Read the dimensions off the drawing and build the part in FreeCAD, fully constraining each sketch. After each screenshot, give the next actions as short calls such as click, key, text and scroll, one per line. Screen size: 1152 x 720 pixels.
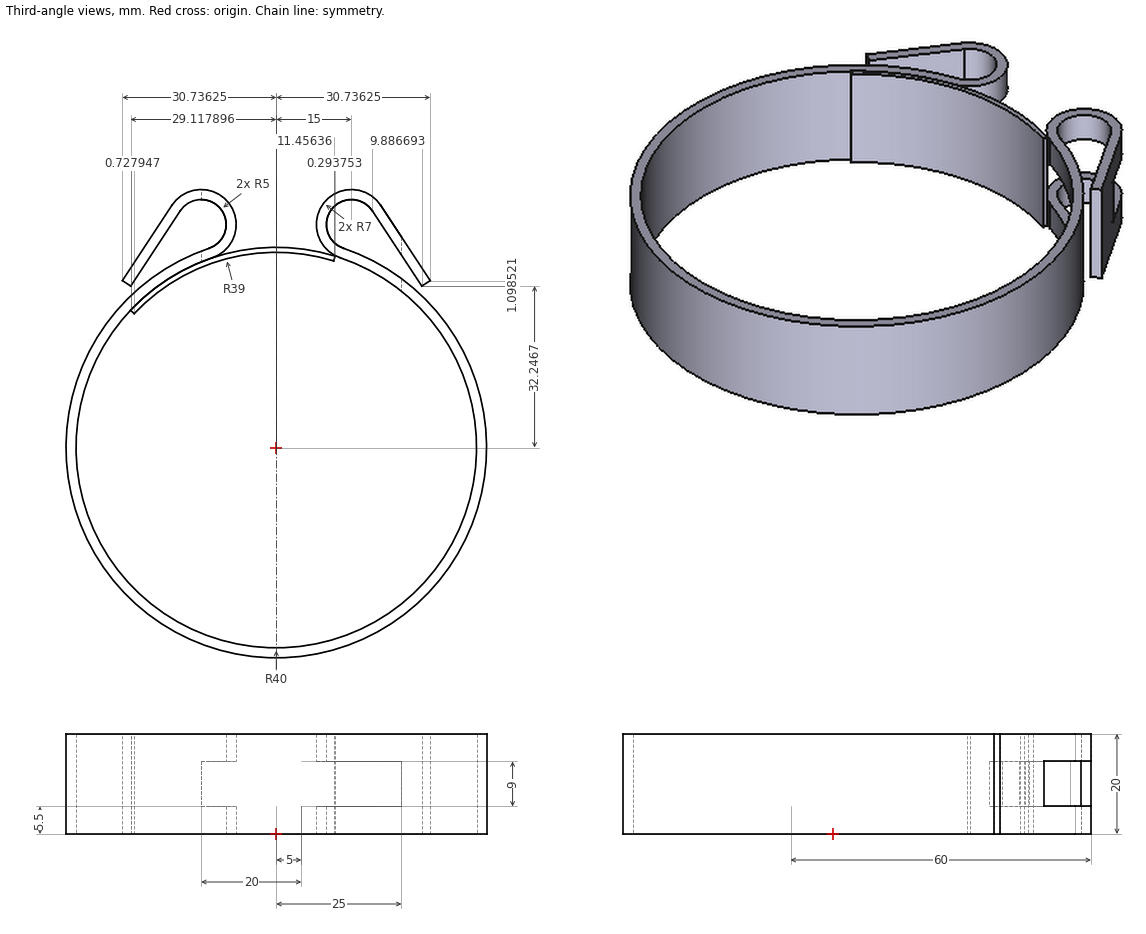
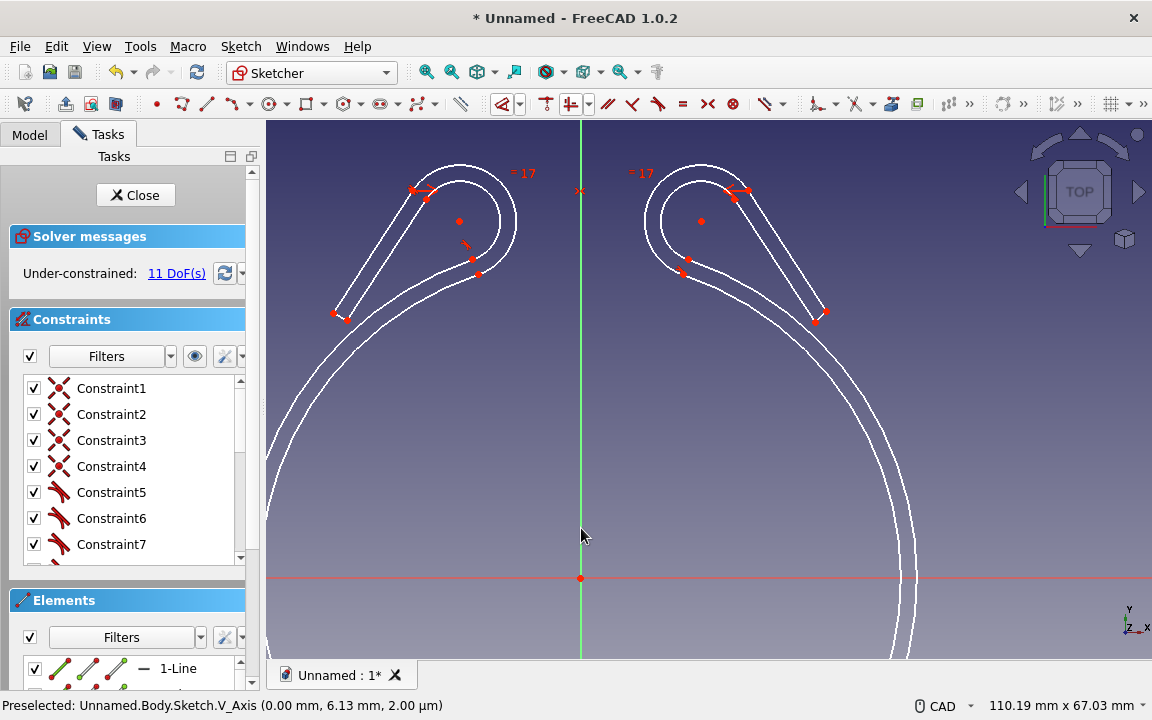
click(815, 322)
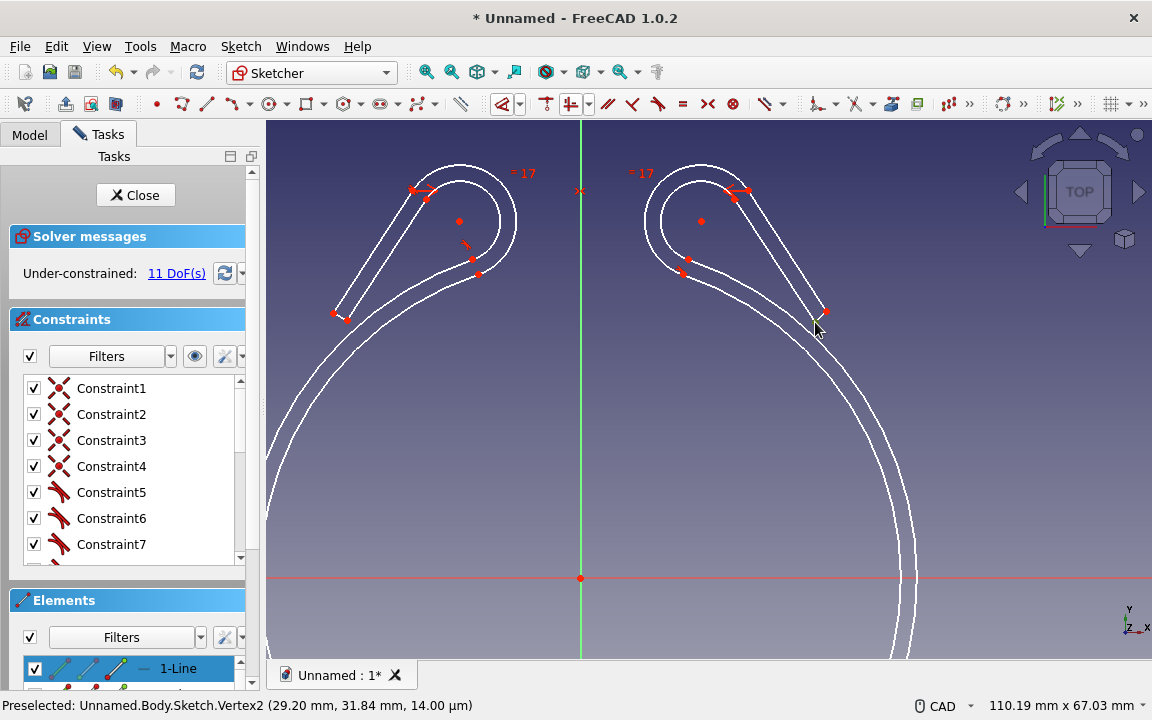
click(347, 320)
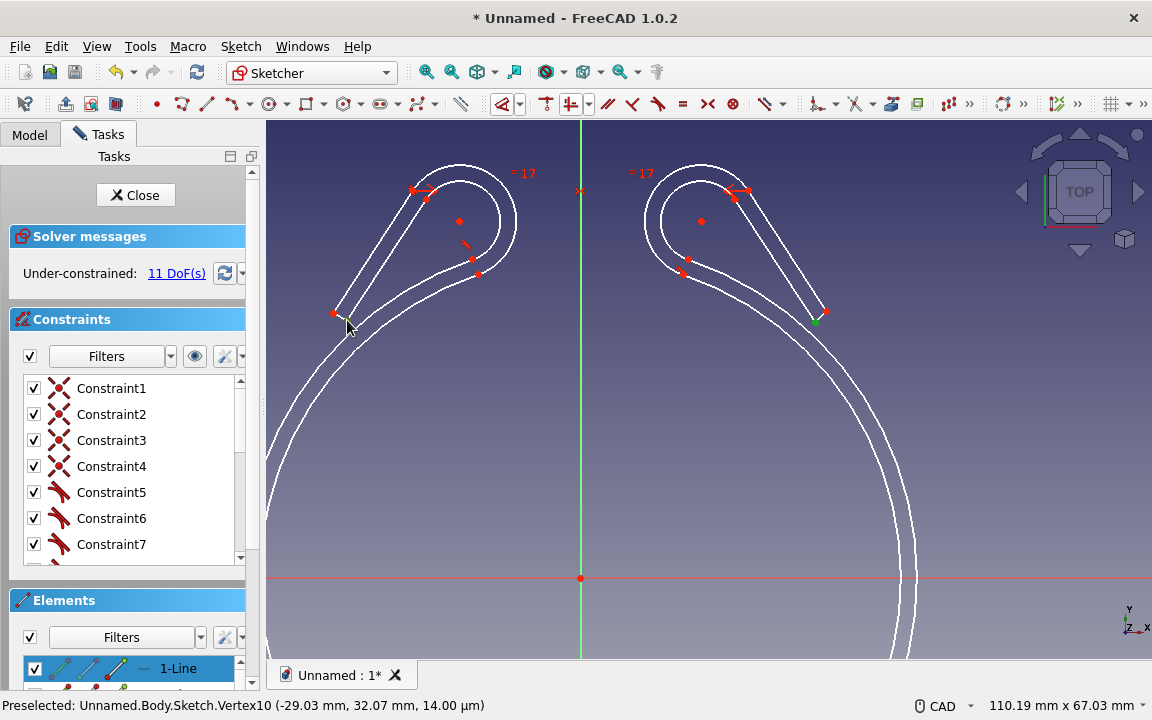
click(581, 528)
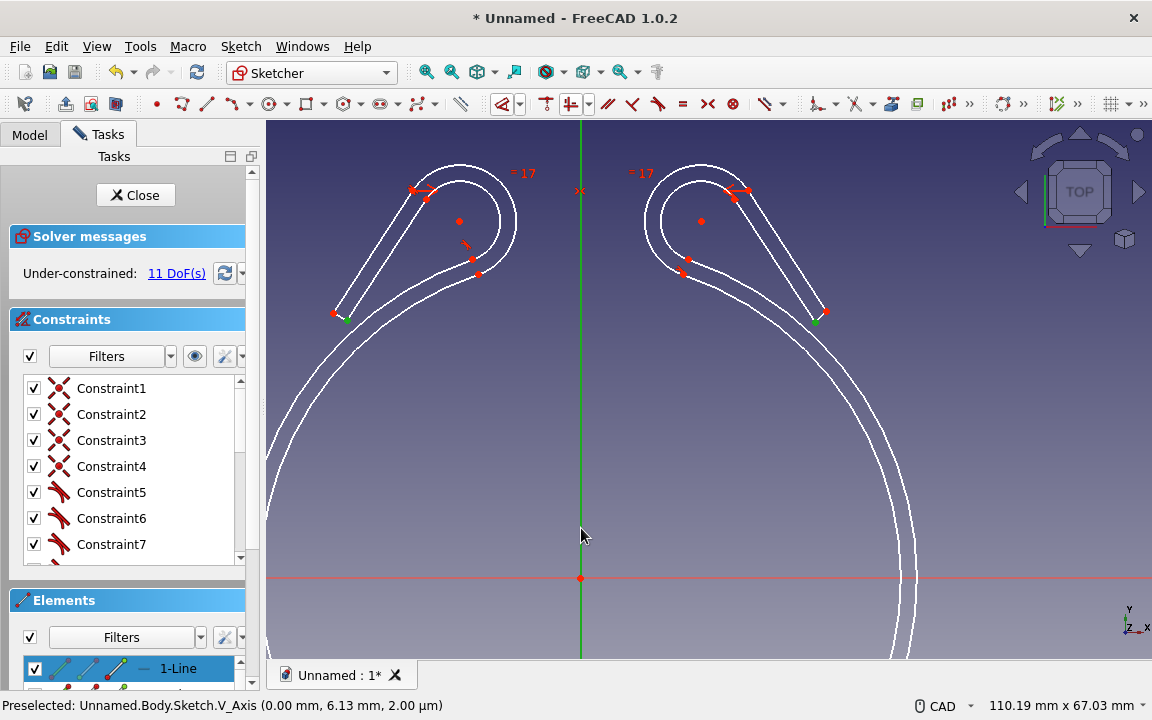
key(s)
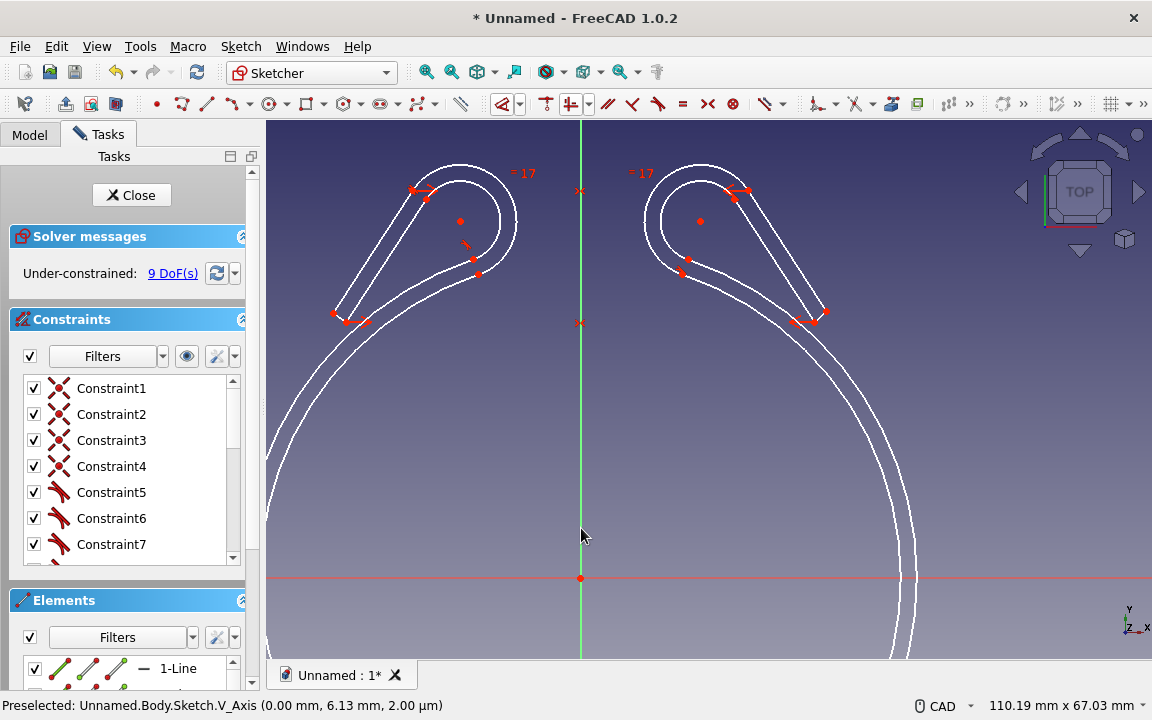
click(693, 166)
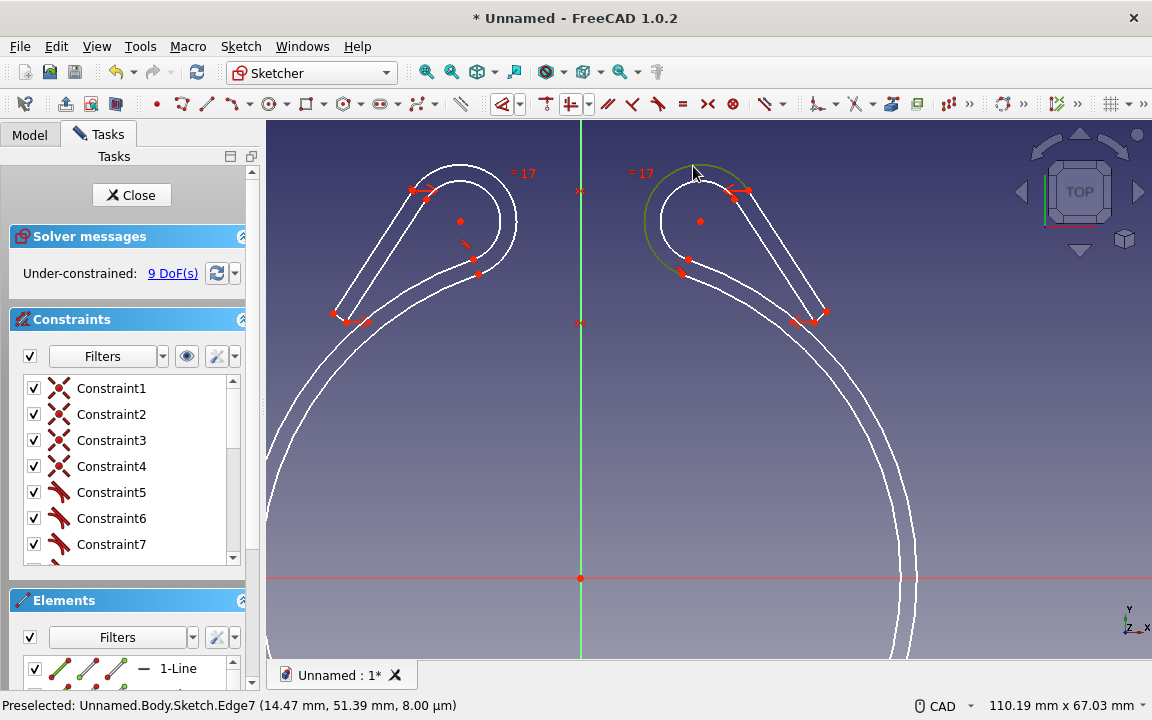
key(k)
key(r)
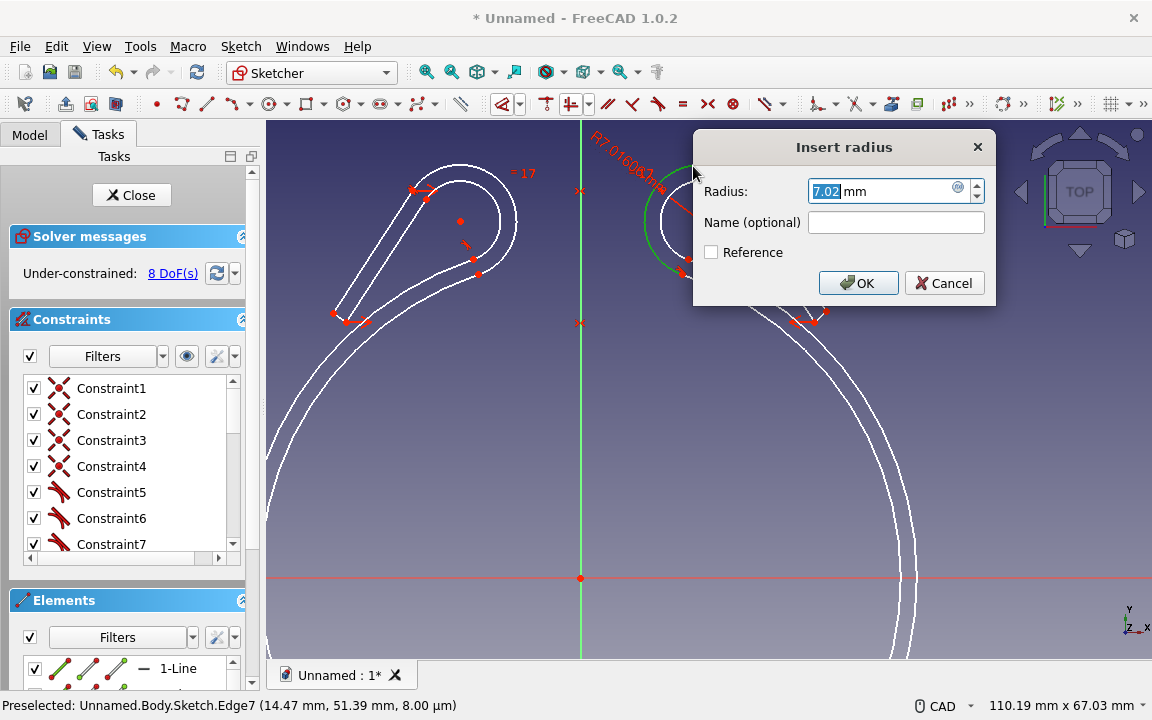
text(7)
key(Return)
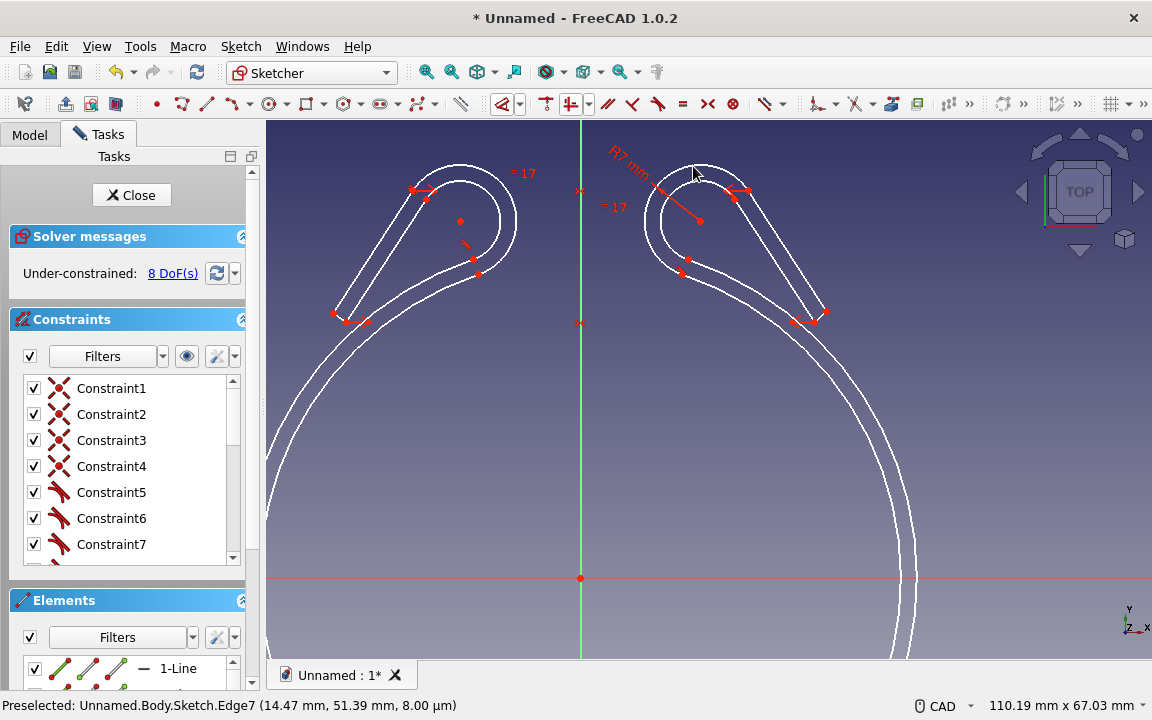
click(899, 540)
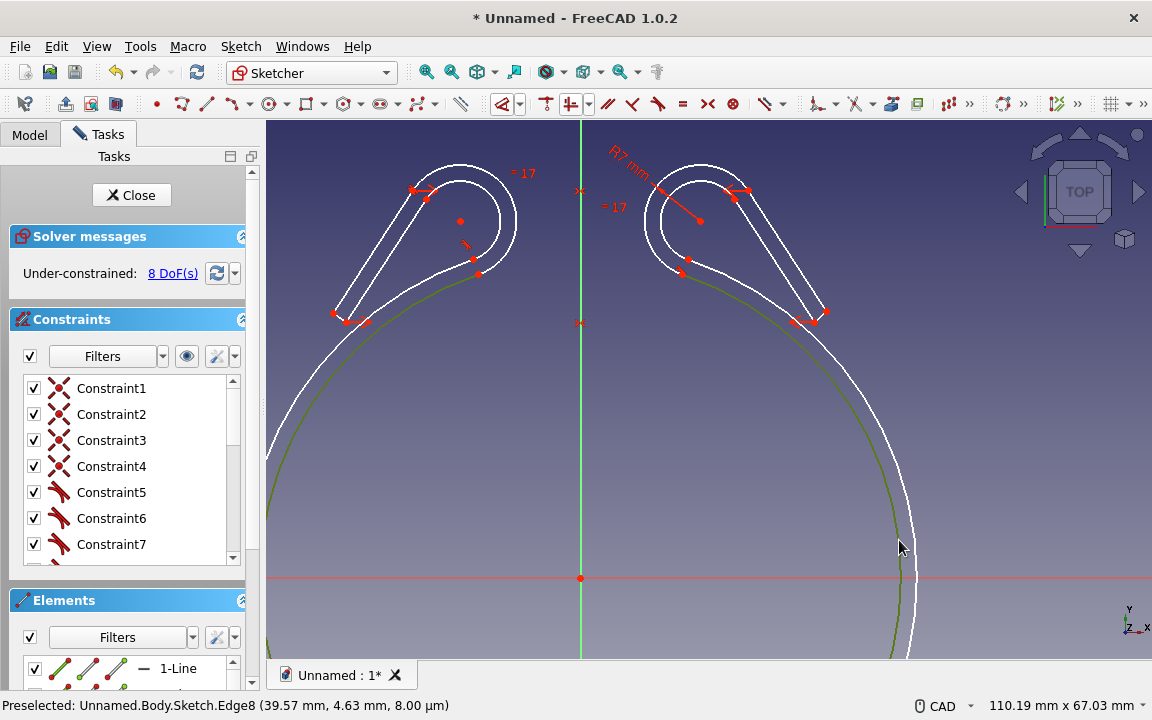
key(k)
key(r)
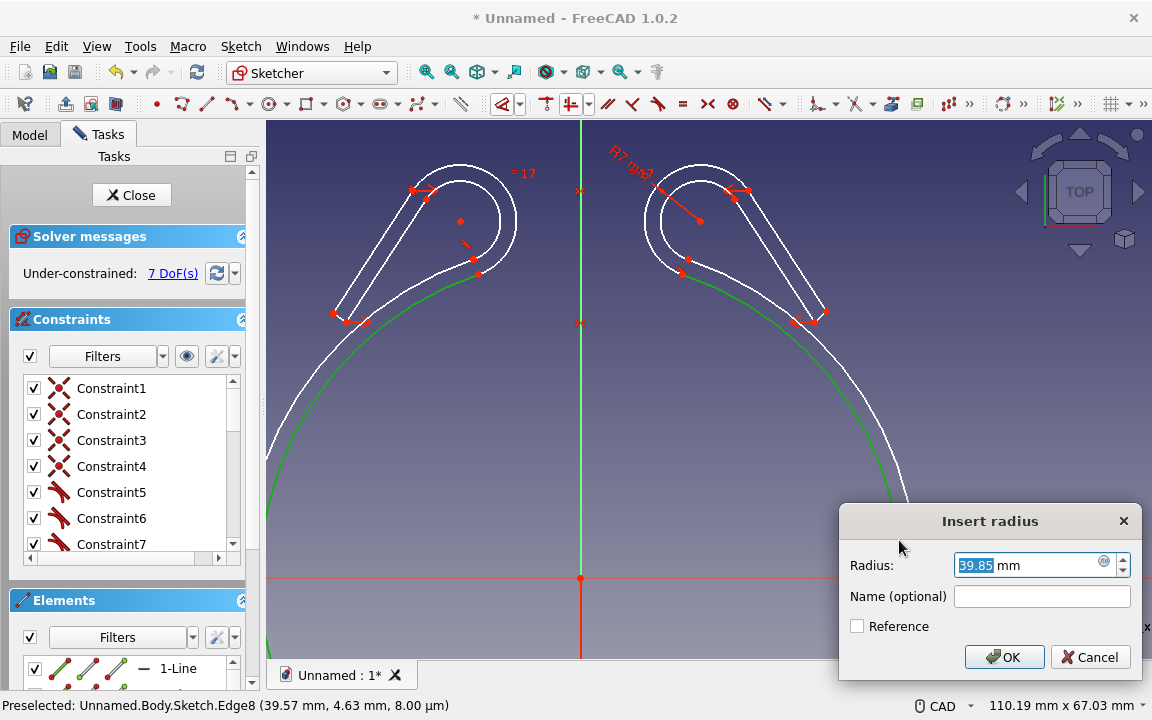
text(40)
key(Return)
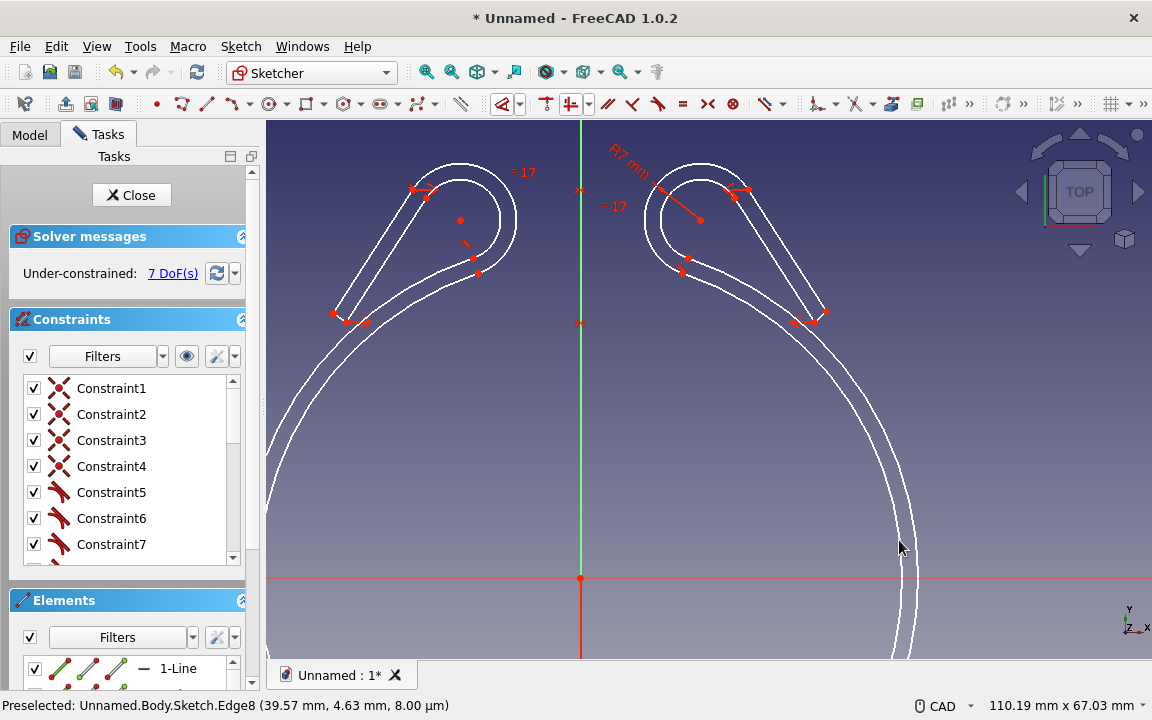
click(500, 224)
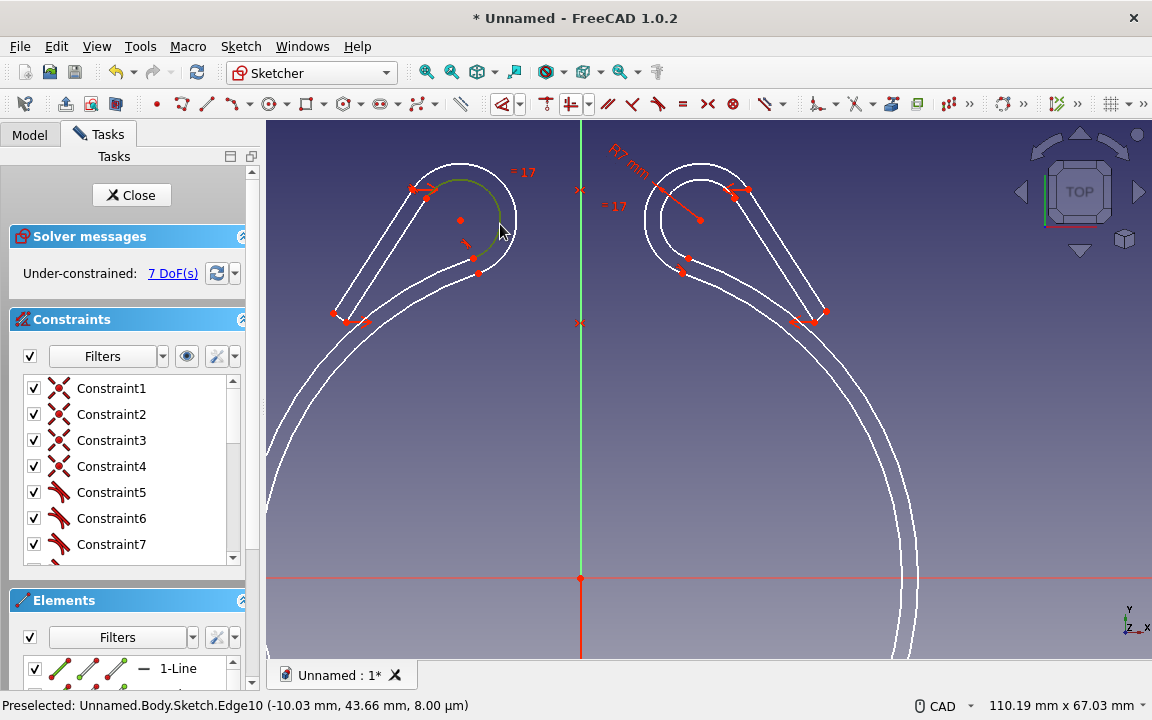
key(k)
key(r)